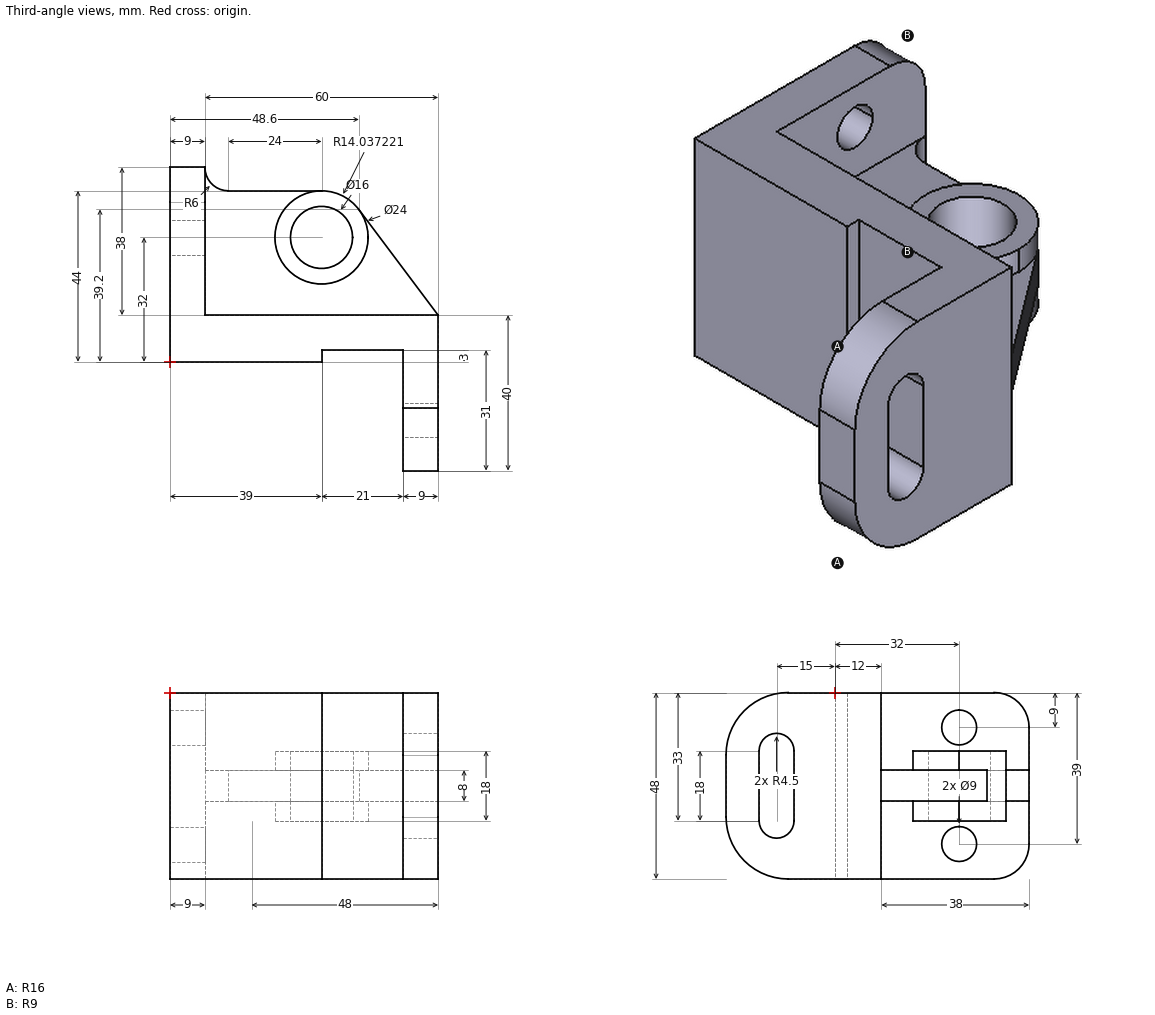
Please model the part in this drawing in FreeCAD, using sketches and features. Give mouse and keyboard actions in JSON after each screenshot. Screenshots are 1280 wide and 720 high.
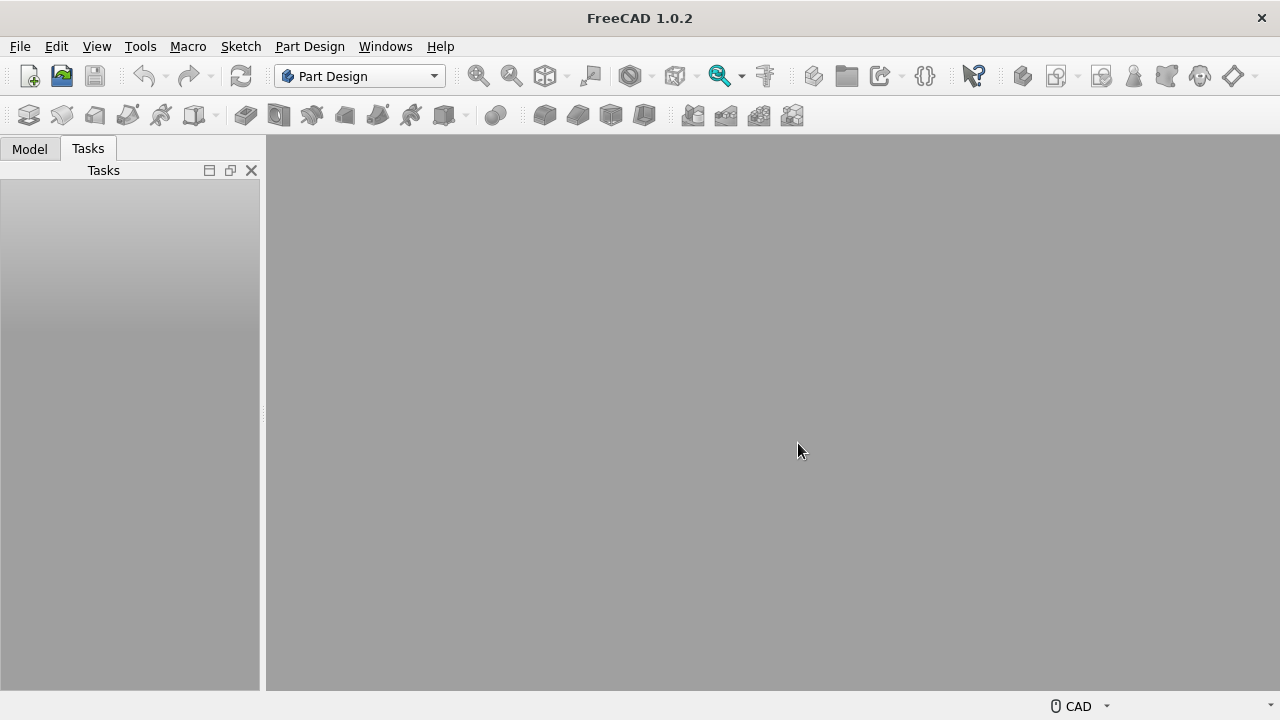
{"action": "key", "text": "ctrl+n"}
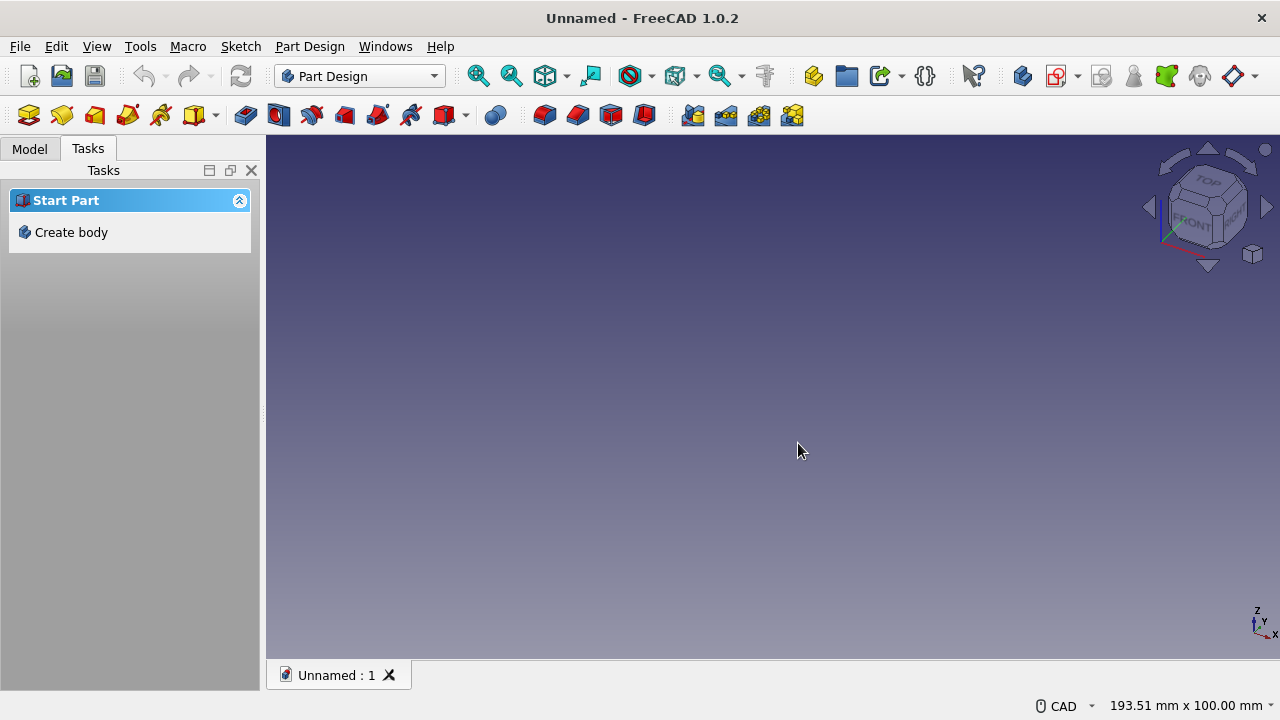
{"action": "left_click", "coordinate": [1056, 76]}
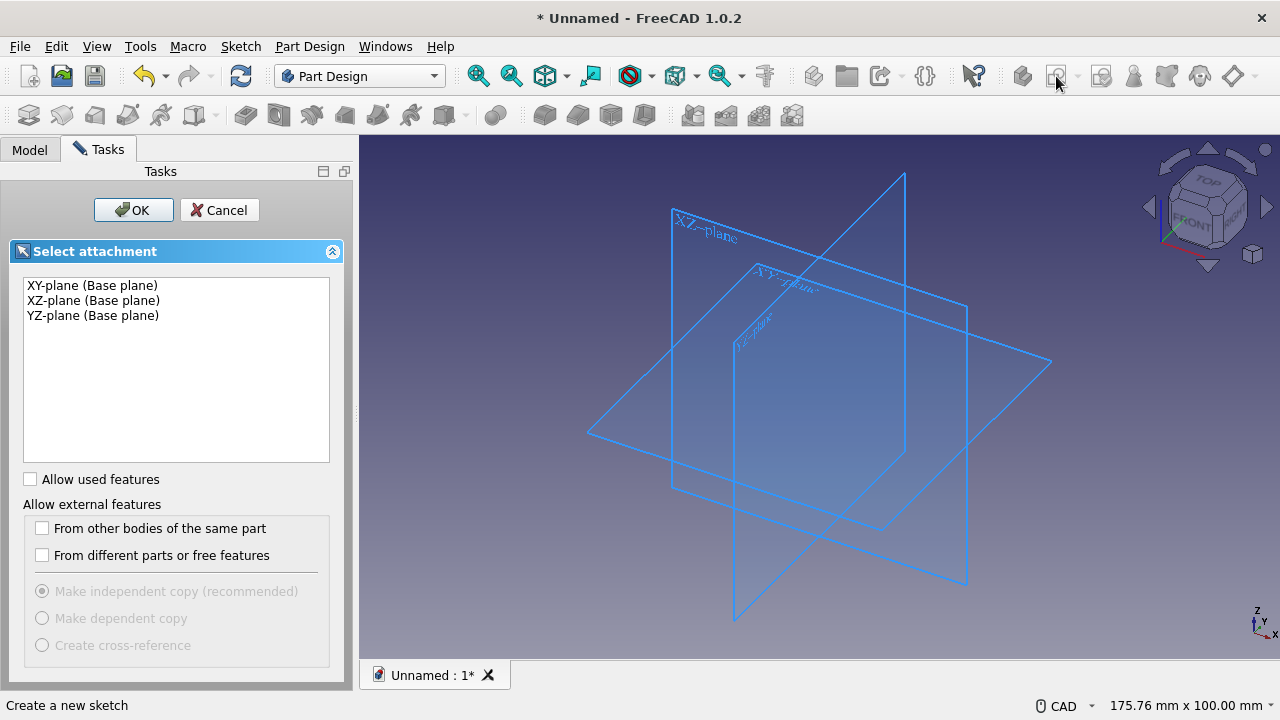
{"action": "left_click", "coordinate": [84, 286]}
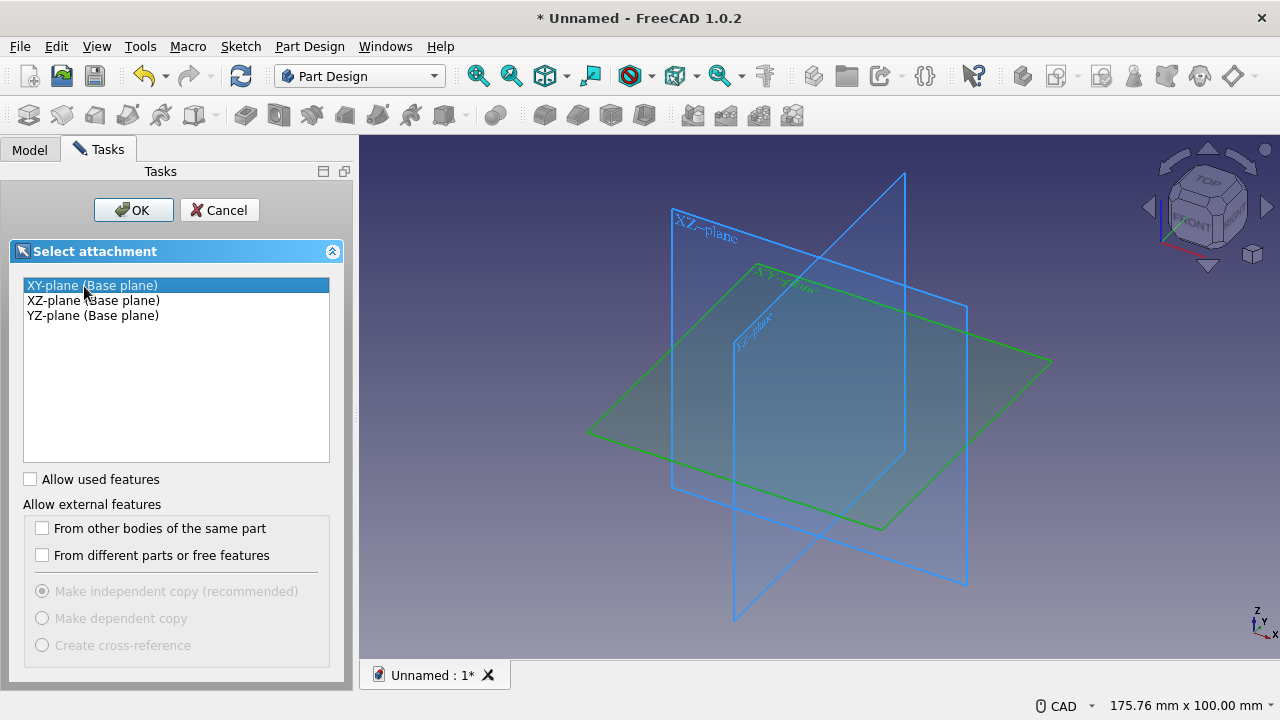
{"action": "left_click", "coordinate": [134, 210]}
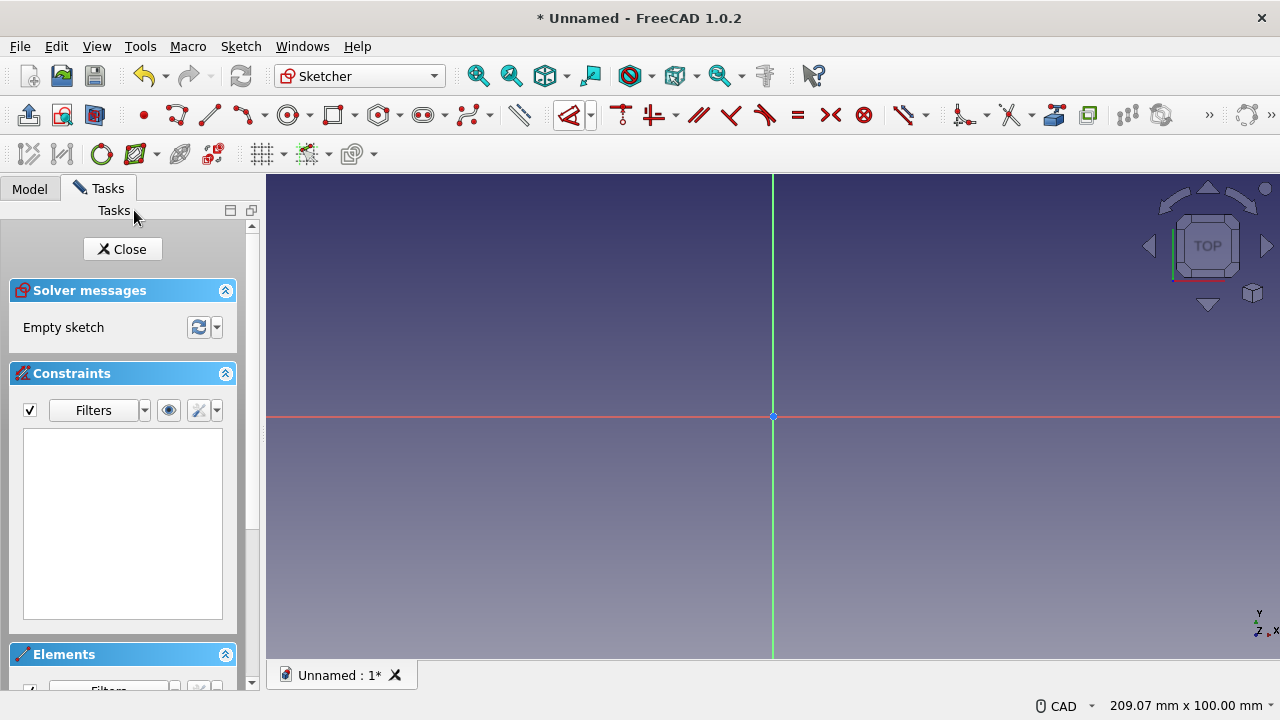
{"action": "scroll", "coordinate": [294, 241], "scroll_direction": "down", "scroll_amount": 1}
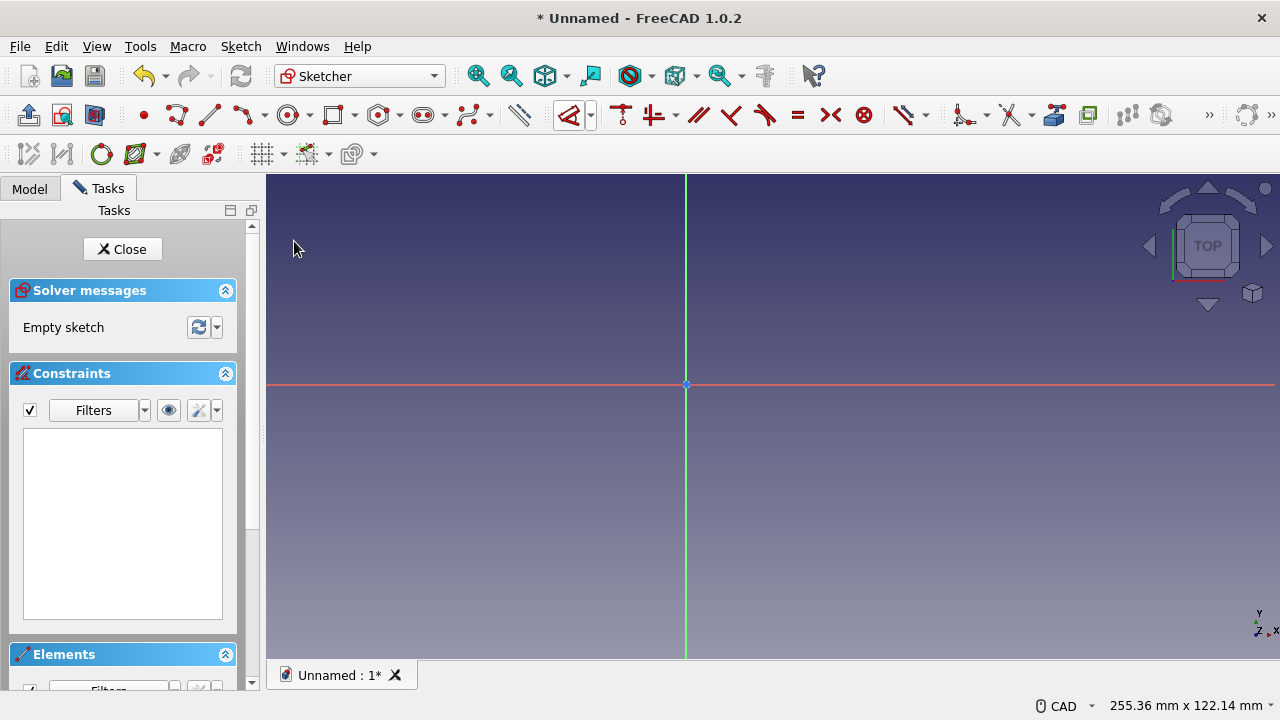
{"action": "scroll", "coordinate": [968, 416], "scroll_direction": "up", "scroll_amount": 3}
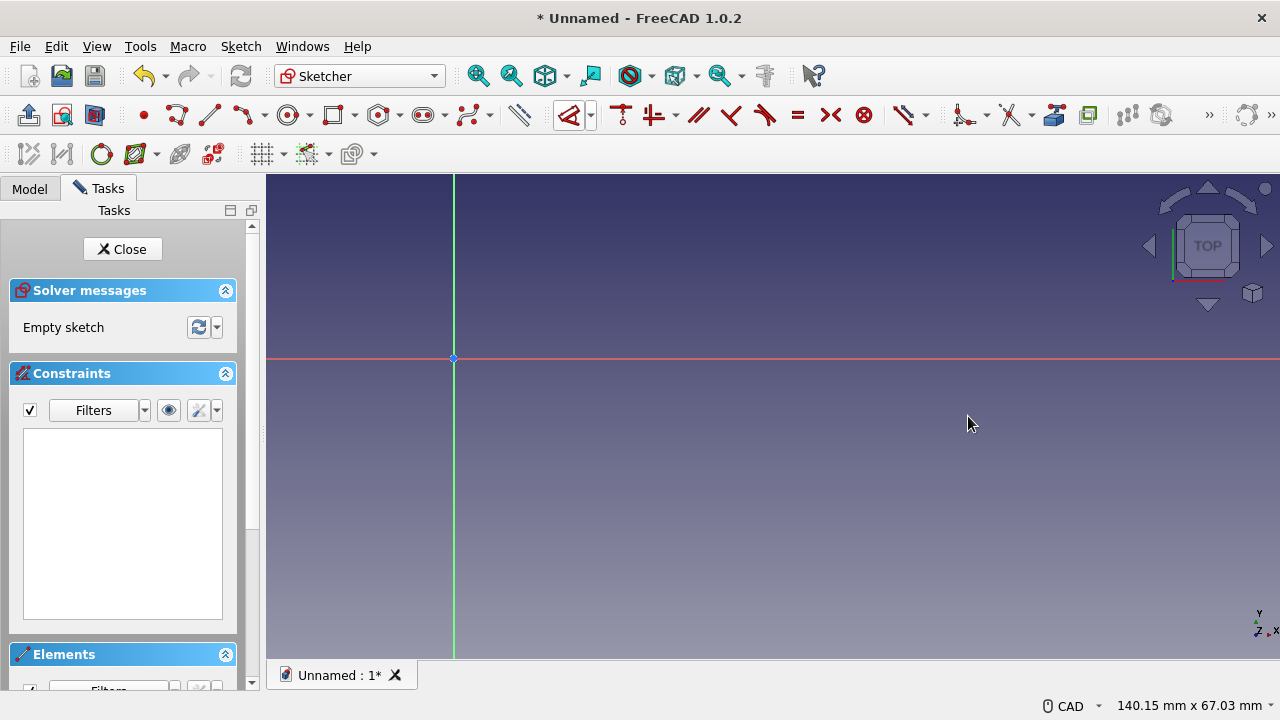
{"action": "key", "text": "g m"}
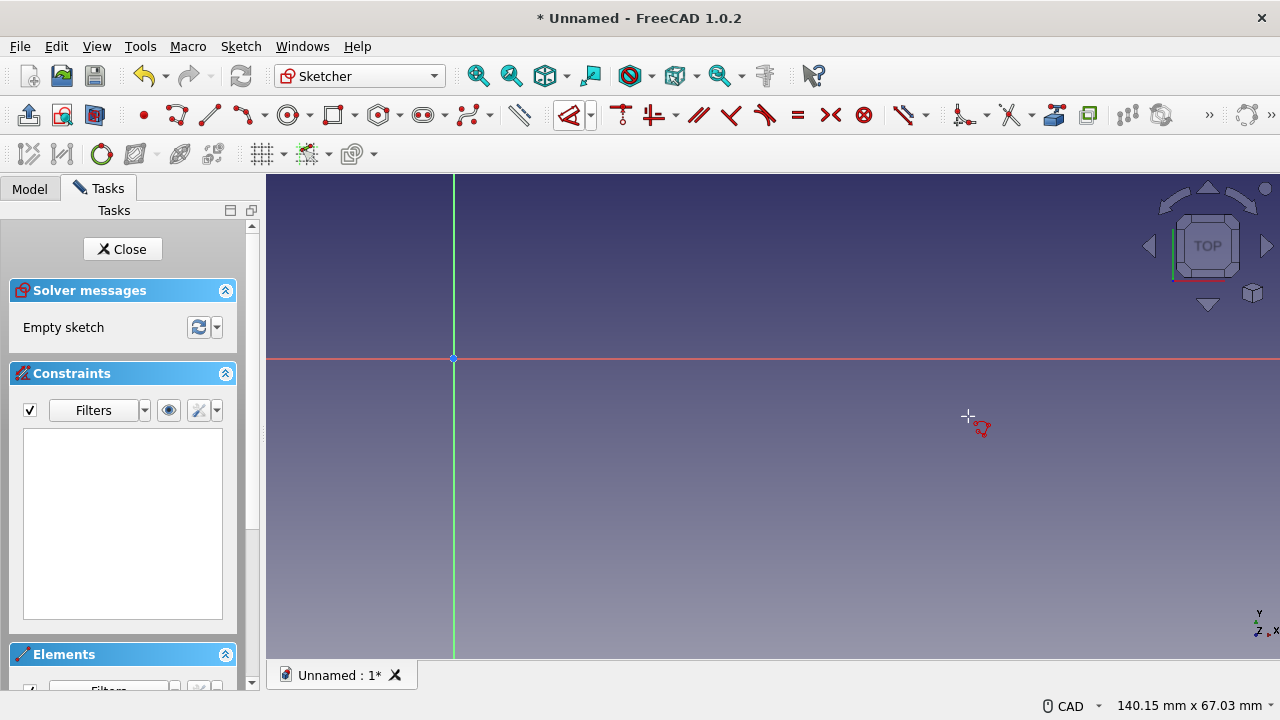
{"action": "left_click", "coordinate": [454, 359]}
{"action": "left_click", "coordinate": [736, 368]}
{"action": "left_click", "coordinate": [736, 337]}
{"action": "left_click", "coordinate": [888, 337]}
{"action": "left_click", "coordinate": [888, 561]}
{"action": "left_click", "coordinate": [953, 561]}
{"action": "left_click", "coordinate": [953, 272]}
{"action": "left_click", "coordinate": [463, 272]}
{"action": "left_click", "coordinate": [454, 359]}
{"action": "key", "text": "Escape"}
{"action": "key", "text": "Escape"}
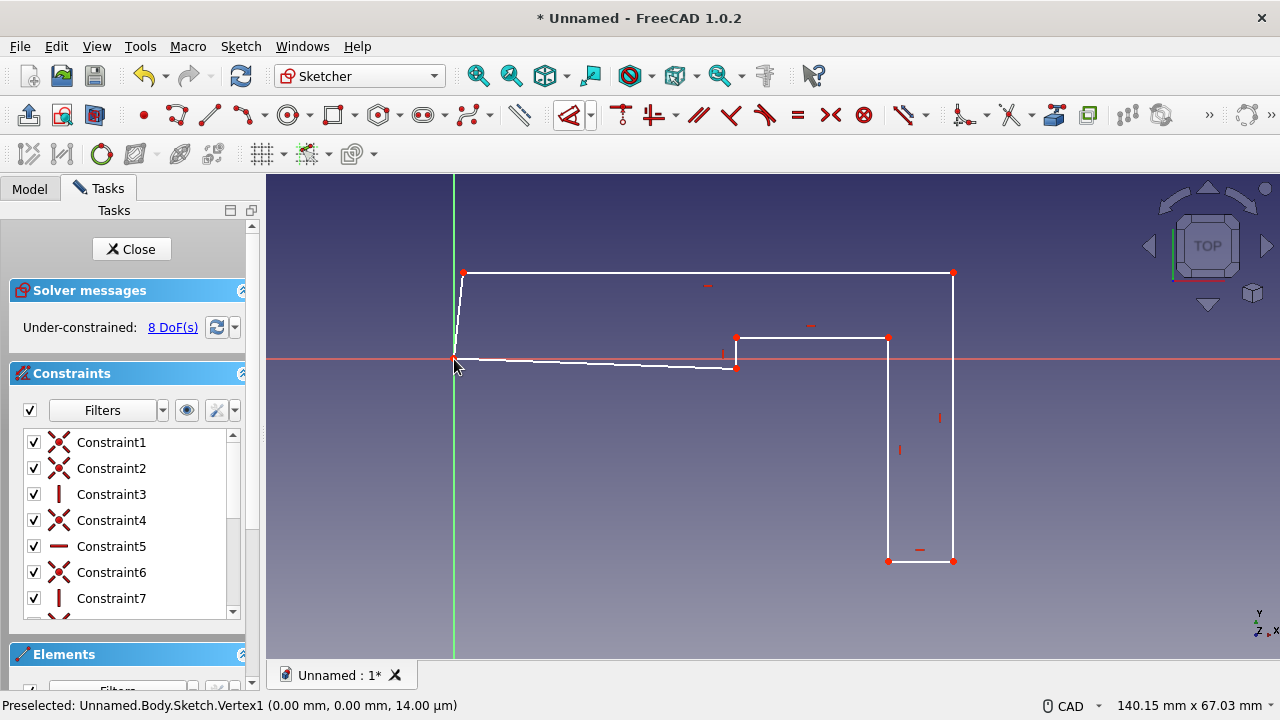
{"action": "left_click", "coordinate": [539, 362]}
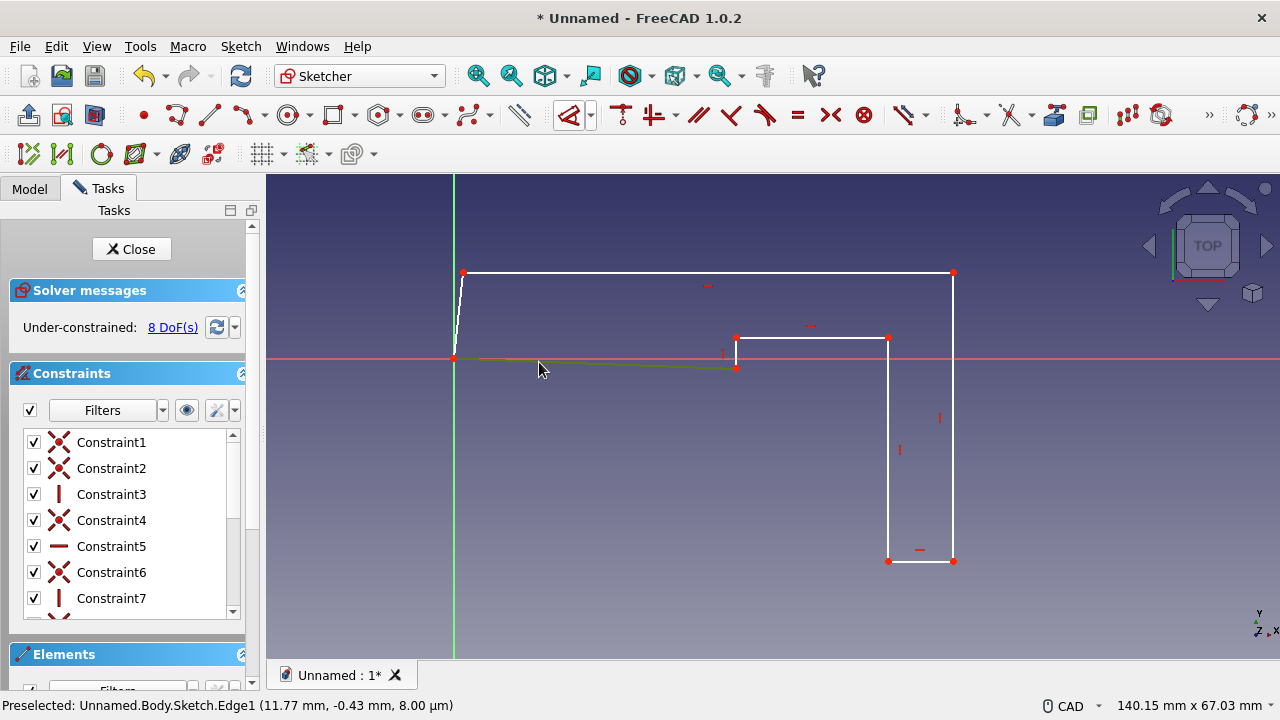
{"action": "left_click", "coordinate": [676, 116]}